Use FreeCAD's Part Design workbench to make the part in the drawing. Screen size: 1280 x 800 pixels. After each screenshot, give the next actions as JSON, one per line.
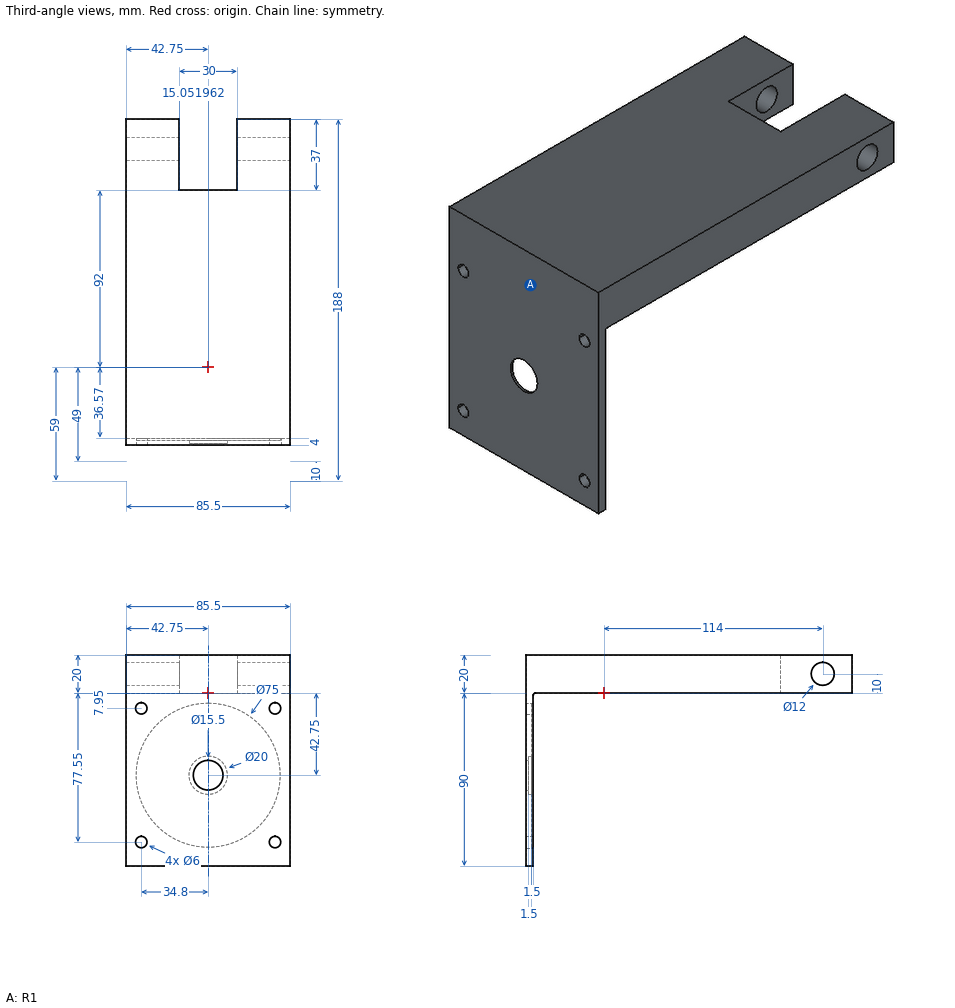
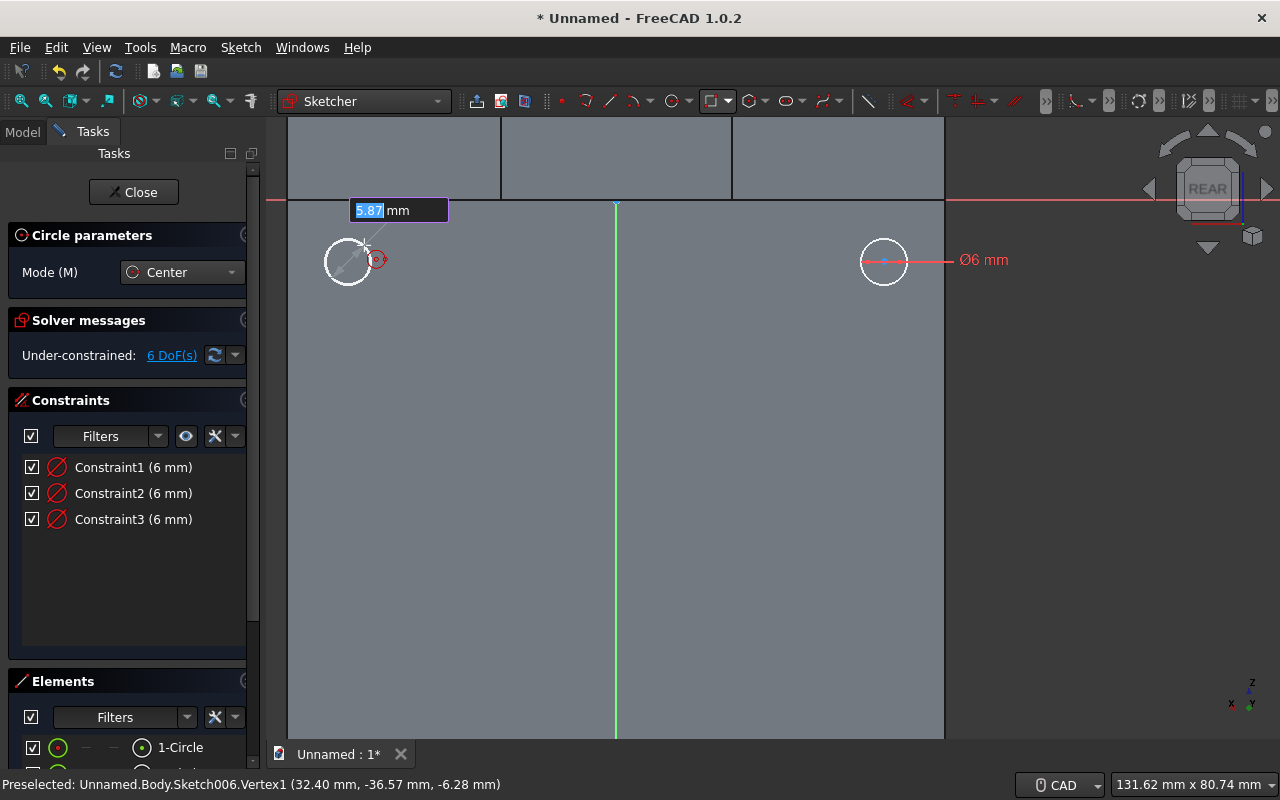
{"action": "type", "text": "6"}
{"action": "key", "text": "Return"}
{"action": "key", "text": "Escape"}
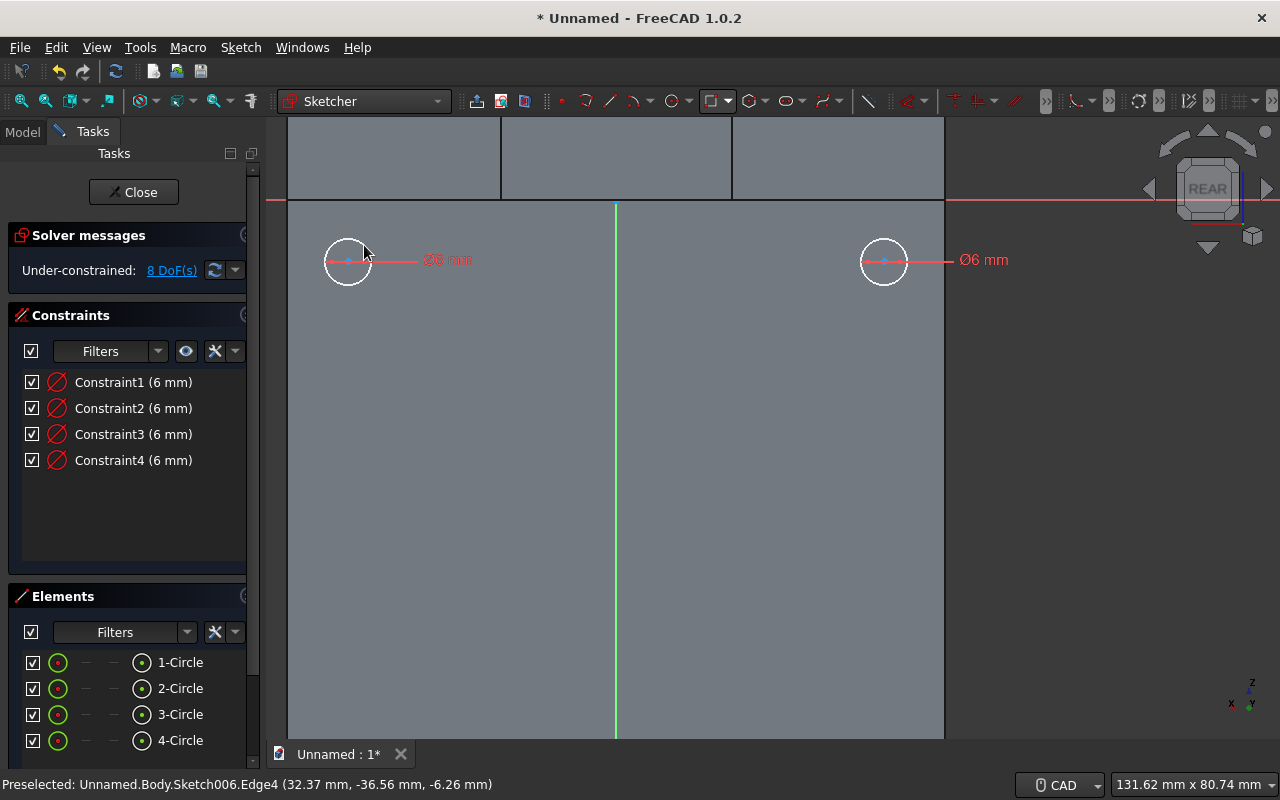
{"action": "scroll", "coordinate": [884, 260], "scroll_direction": "down", "scroll_amount": 2}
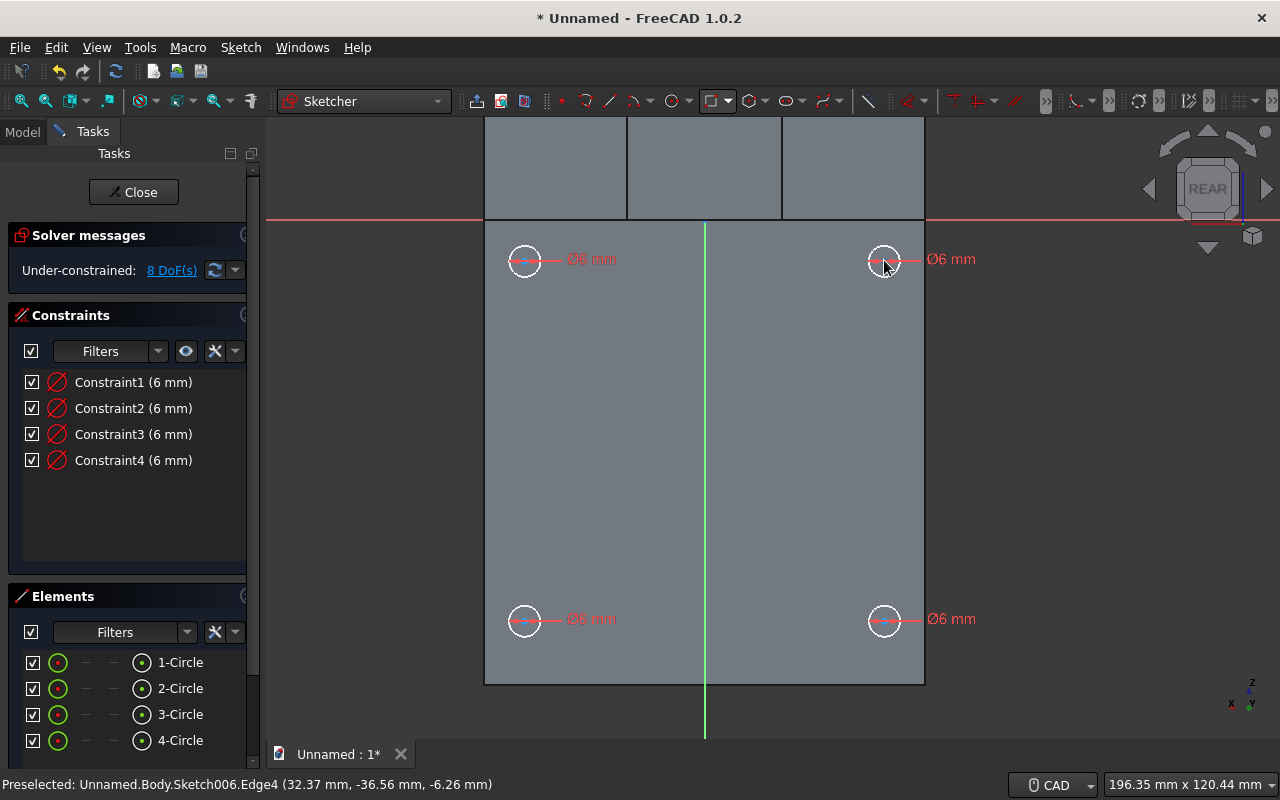
{"action": "left_click", "coordinate": [885, 621]}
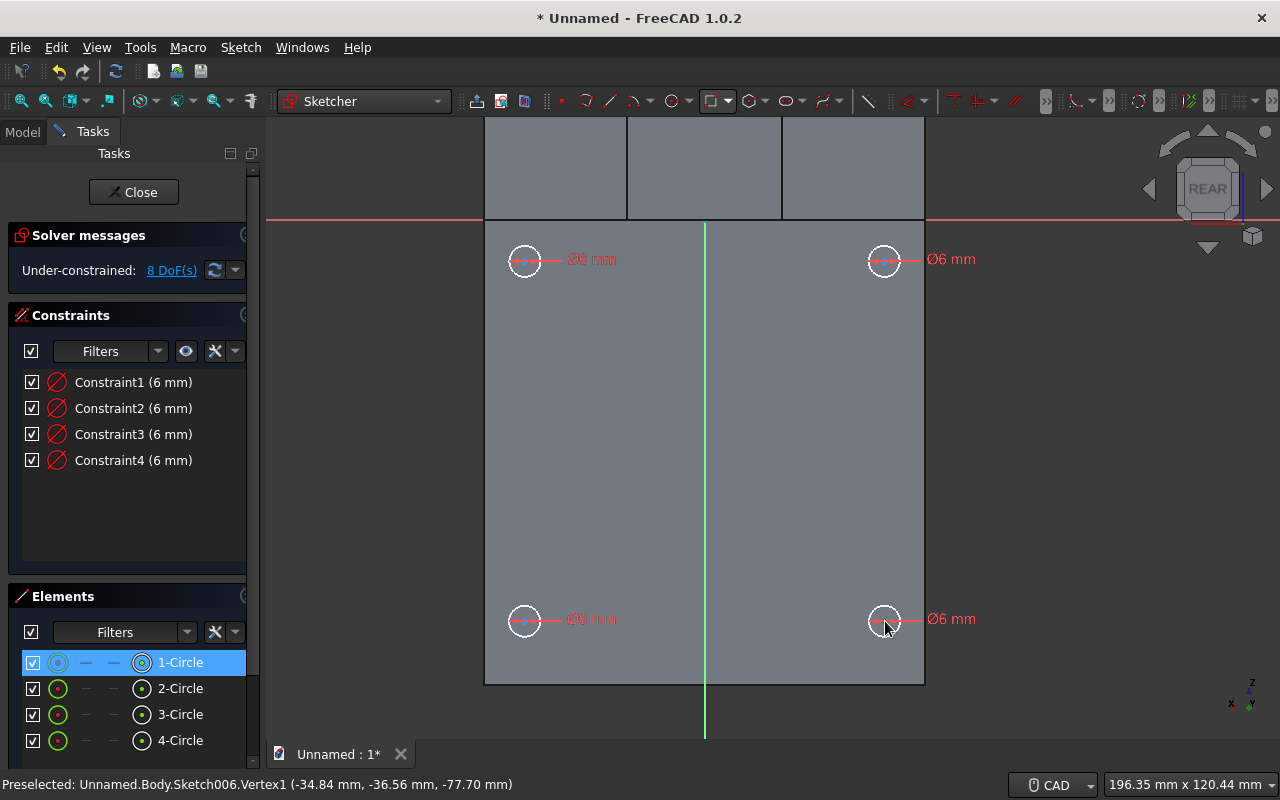
{"action": "left_click", "coordinate": [525, 621]}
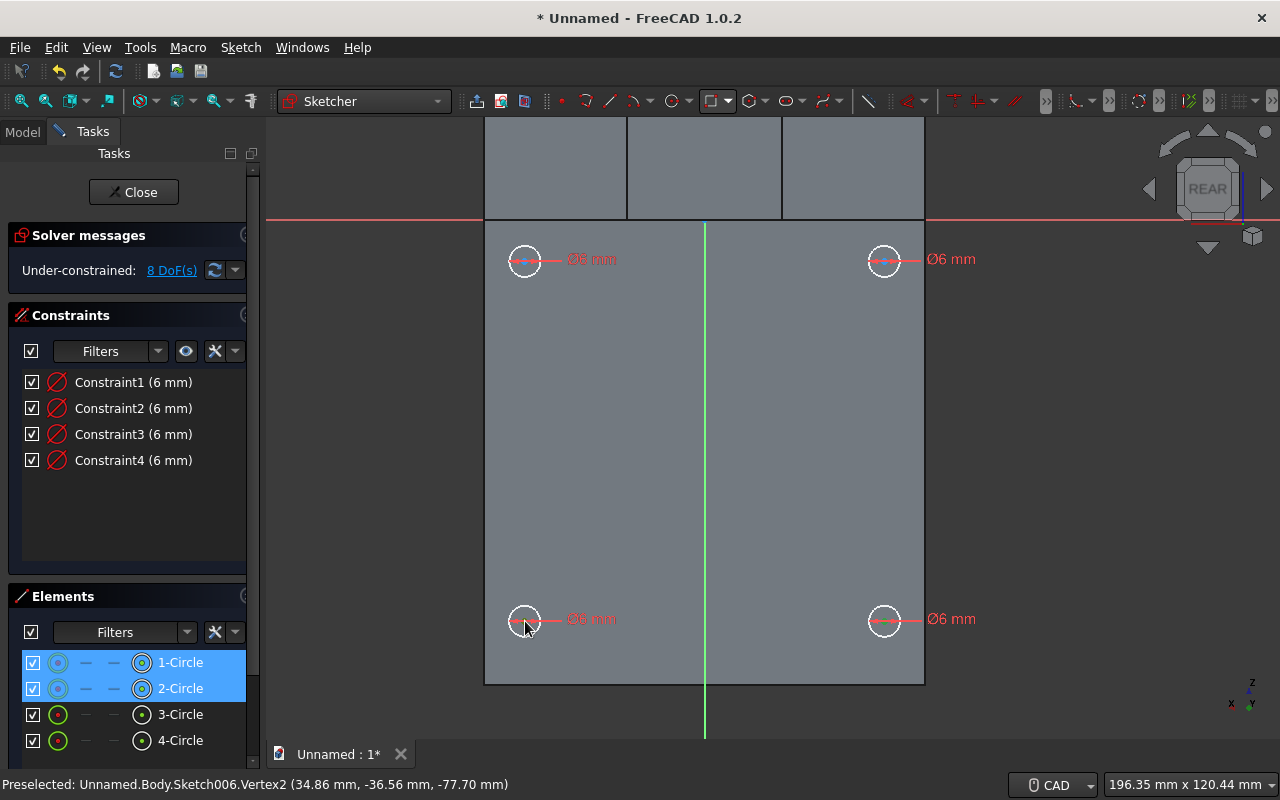
{"action": "left_click", "coordinate": [705, 671]}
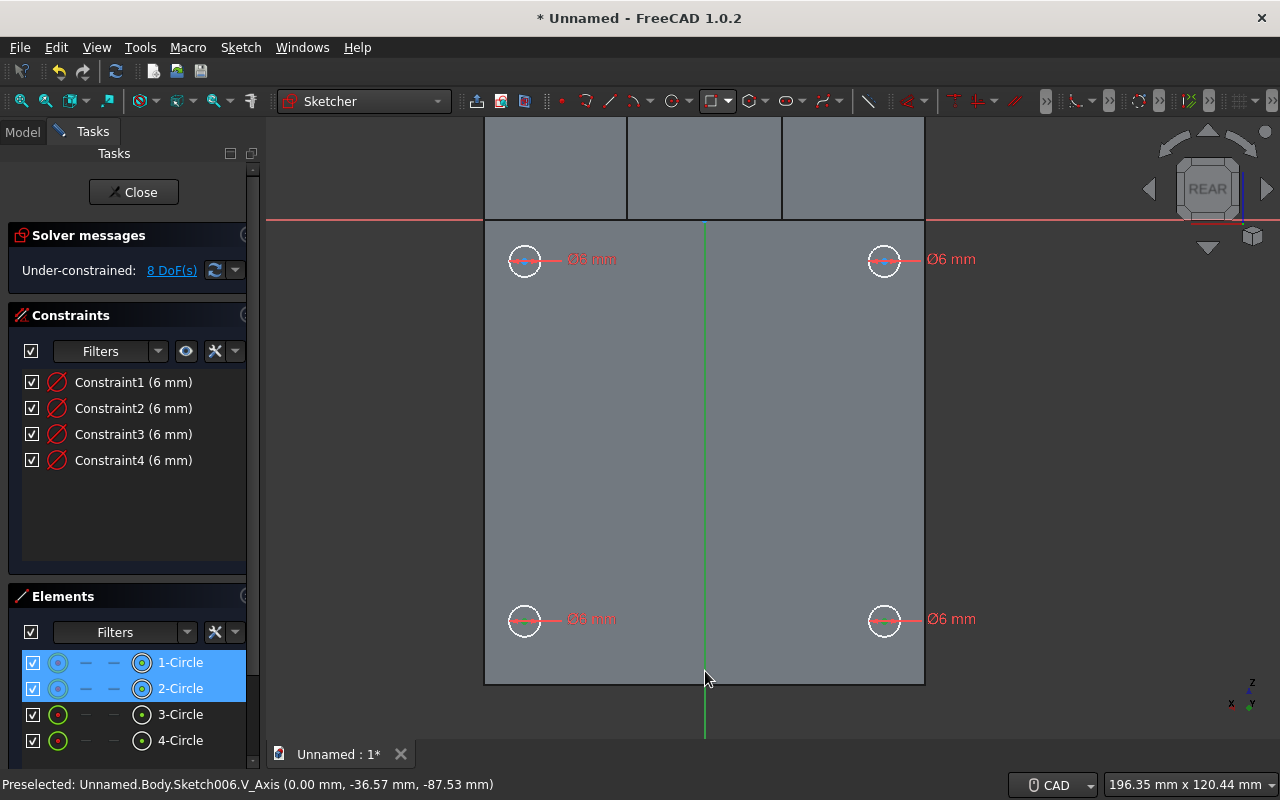
{"action": "key", "text": "s"}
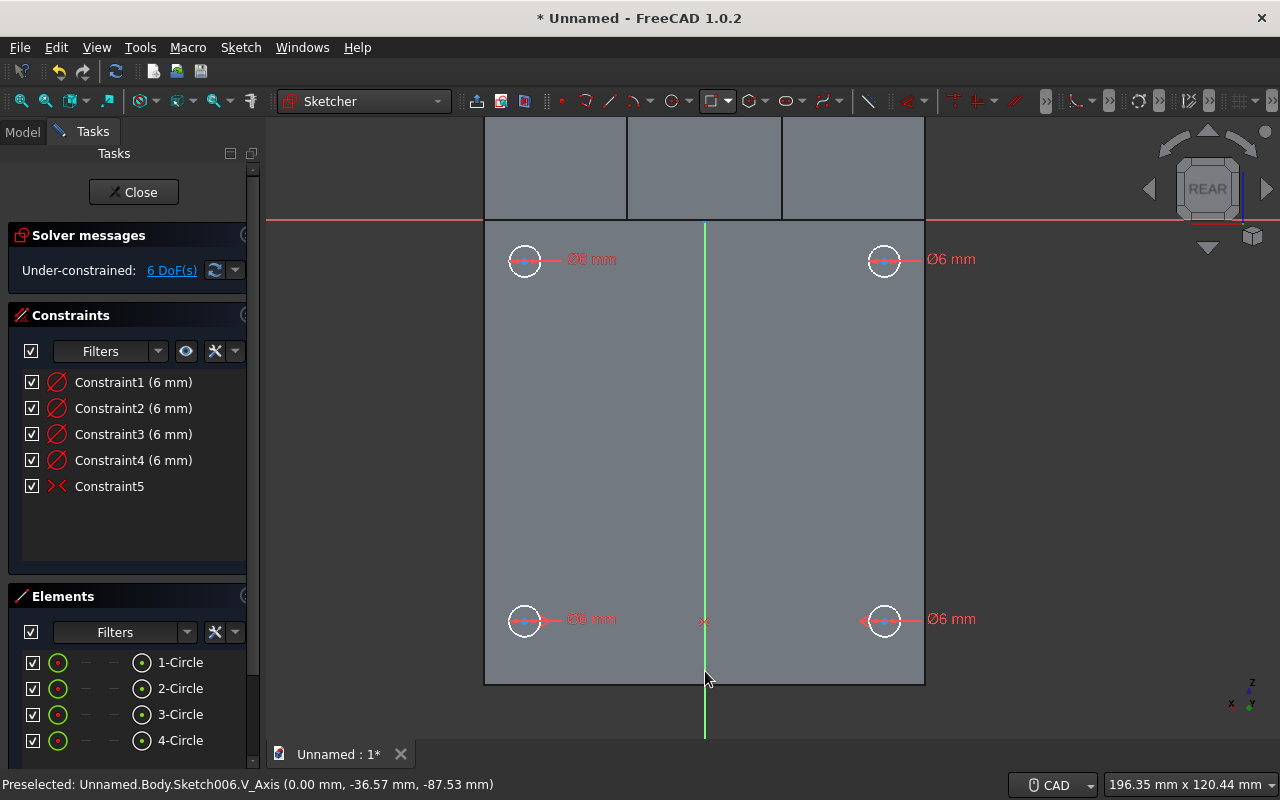
{"action": "left_click", "coordinate": [884, 261]}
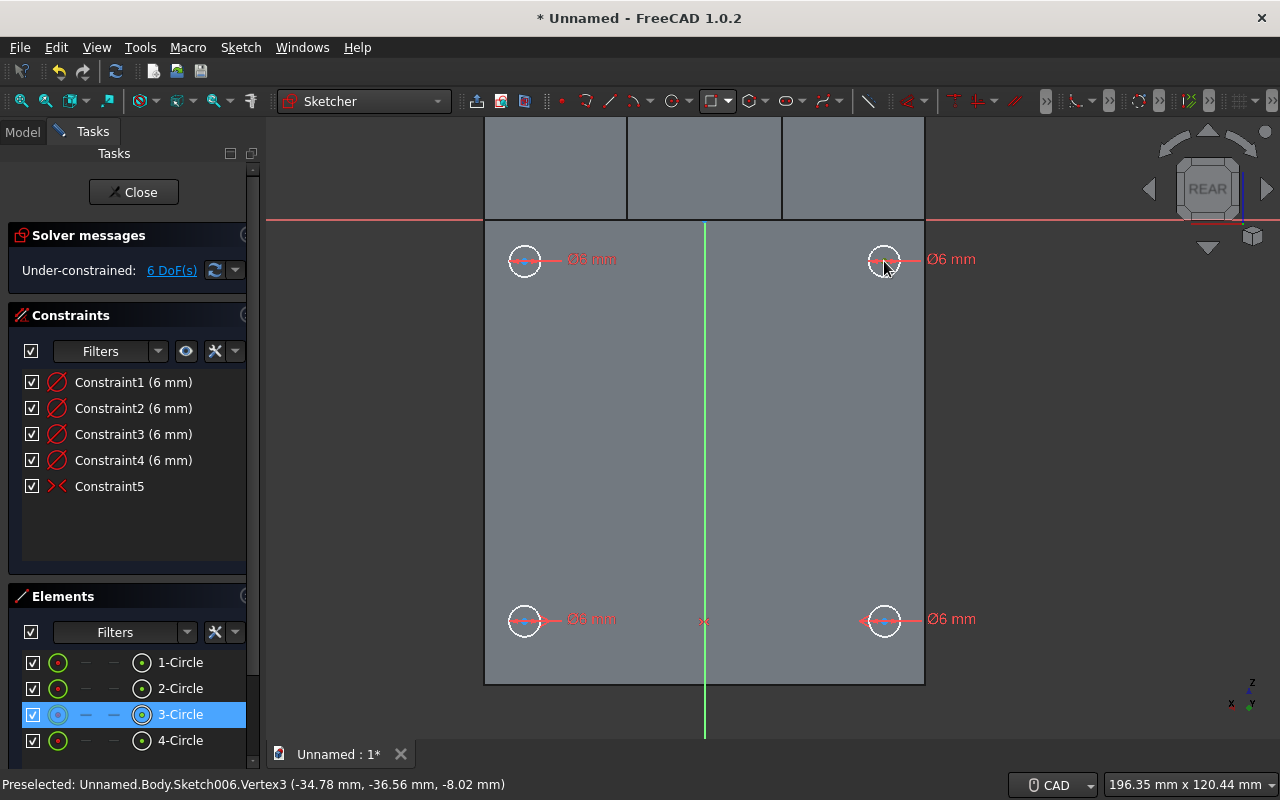
{"action": "left_click", "coordinate": [525, 261]}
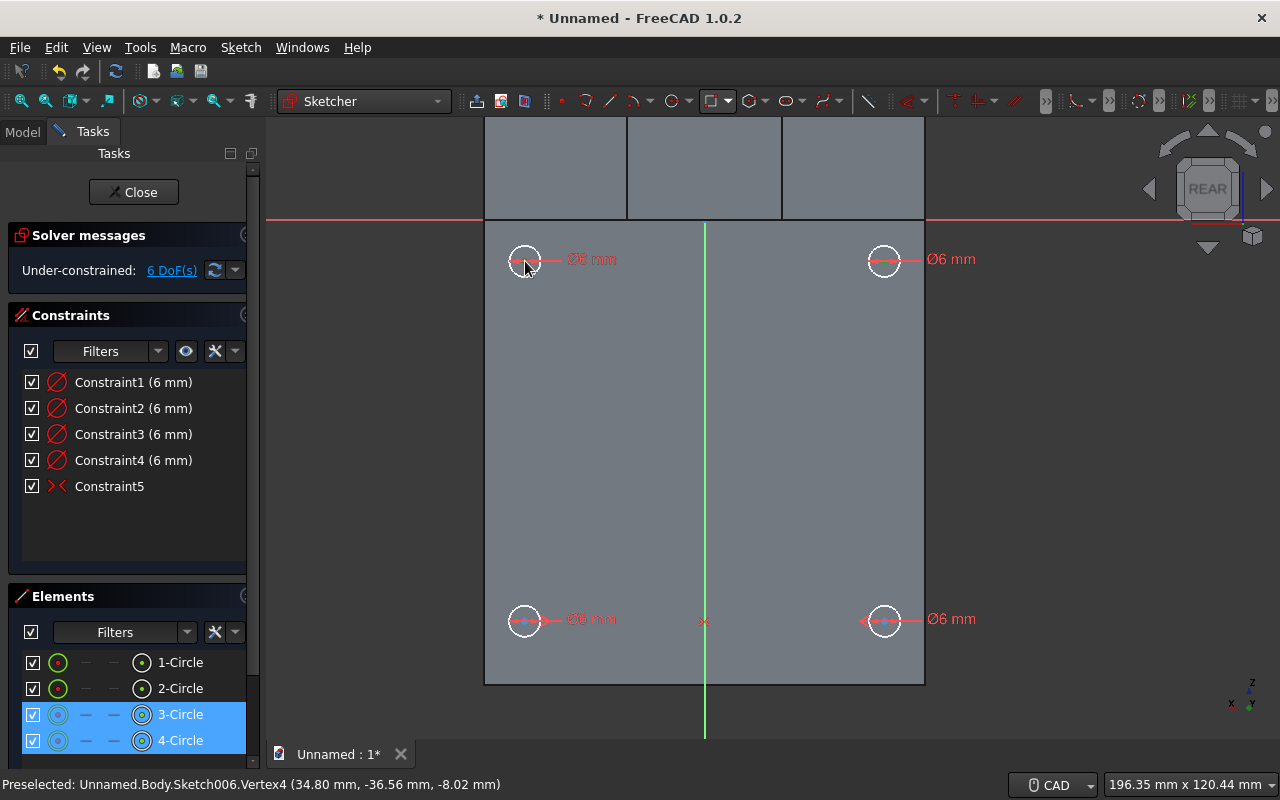
{"action": "left_click", "coordinate": [705, 671]}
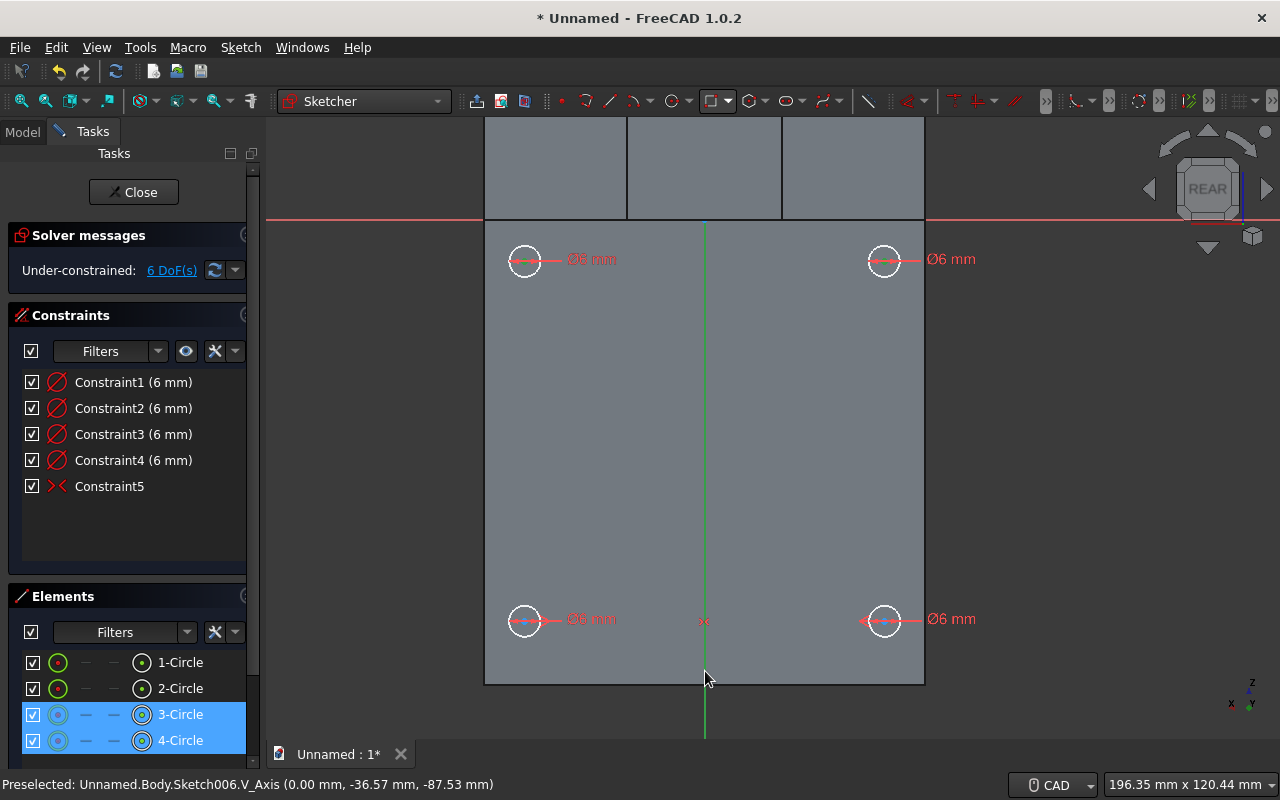
{"action": "key", "text": "s"}